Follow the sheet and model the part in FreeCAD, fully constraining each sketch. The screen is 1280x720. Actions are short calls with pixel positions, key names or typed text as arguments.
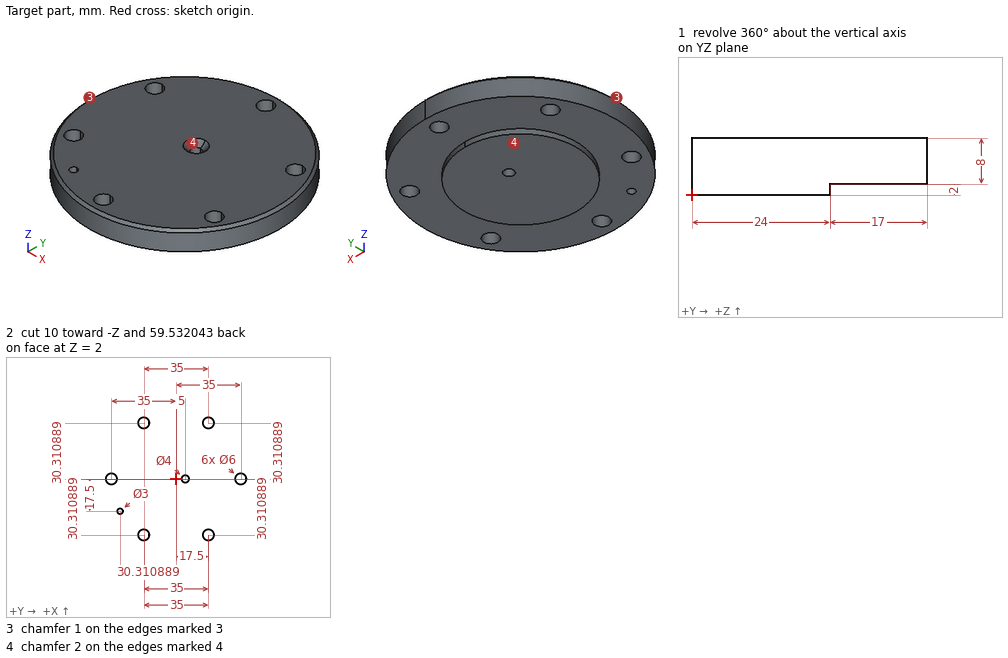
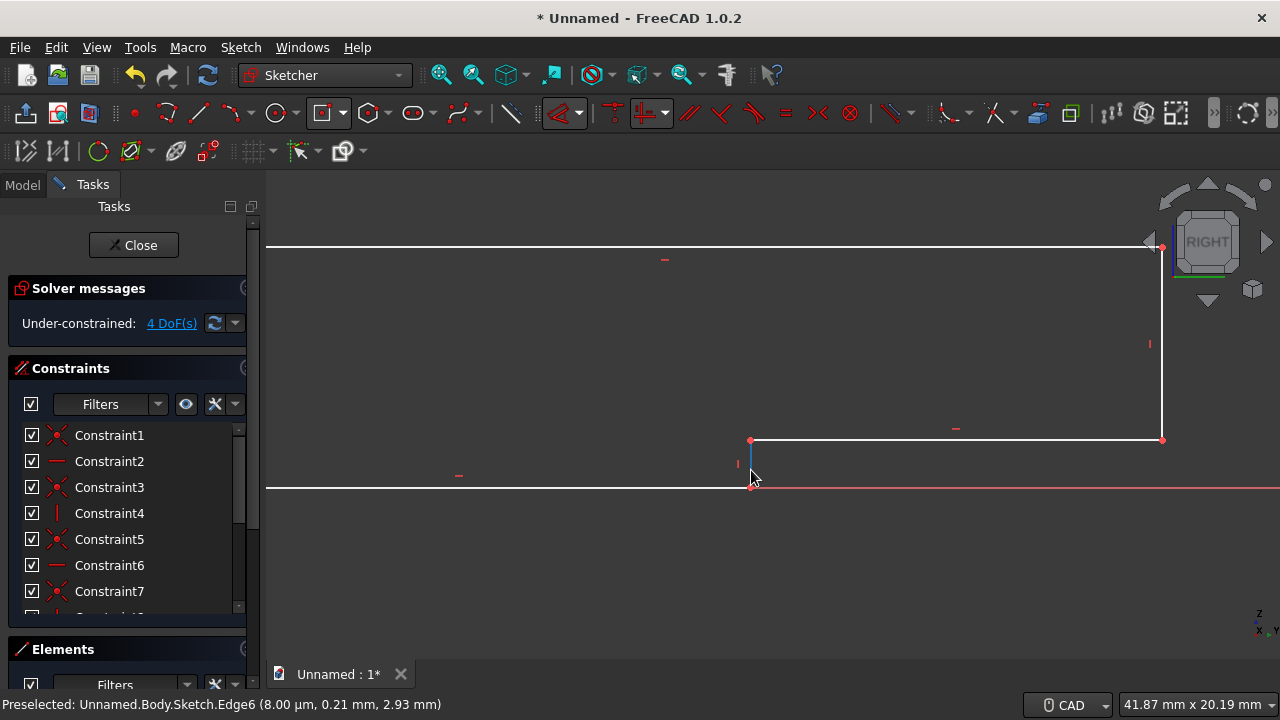
click(751, 469)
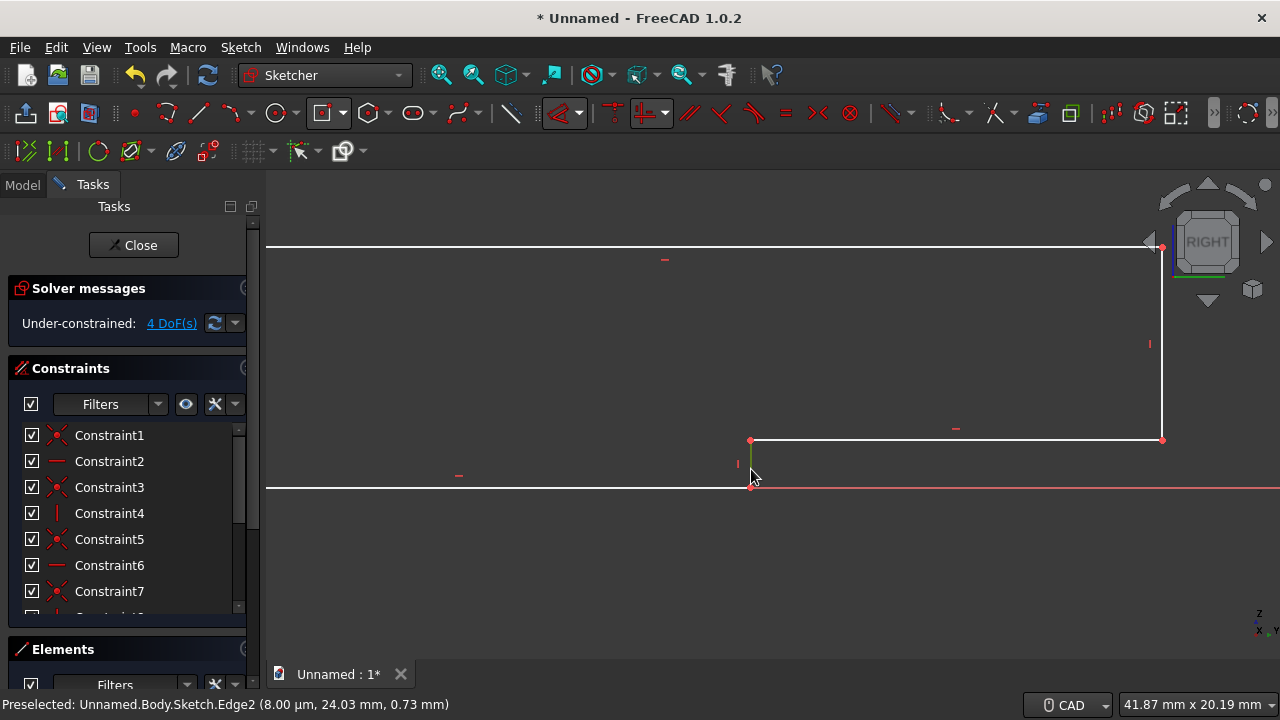
key(i)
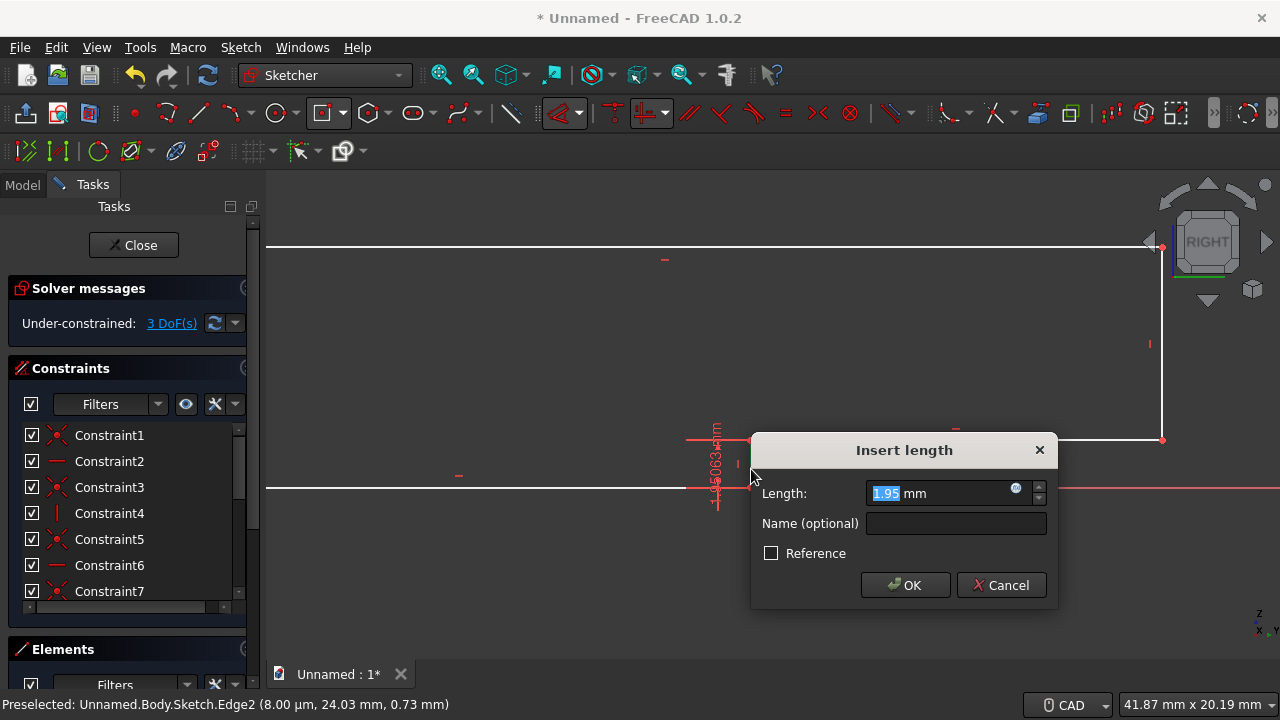
text(2)
key(Return)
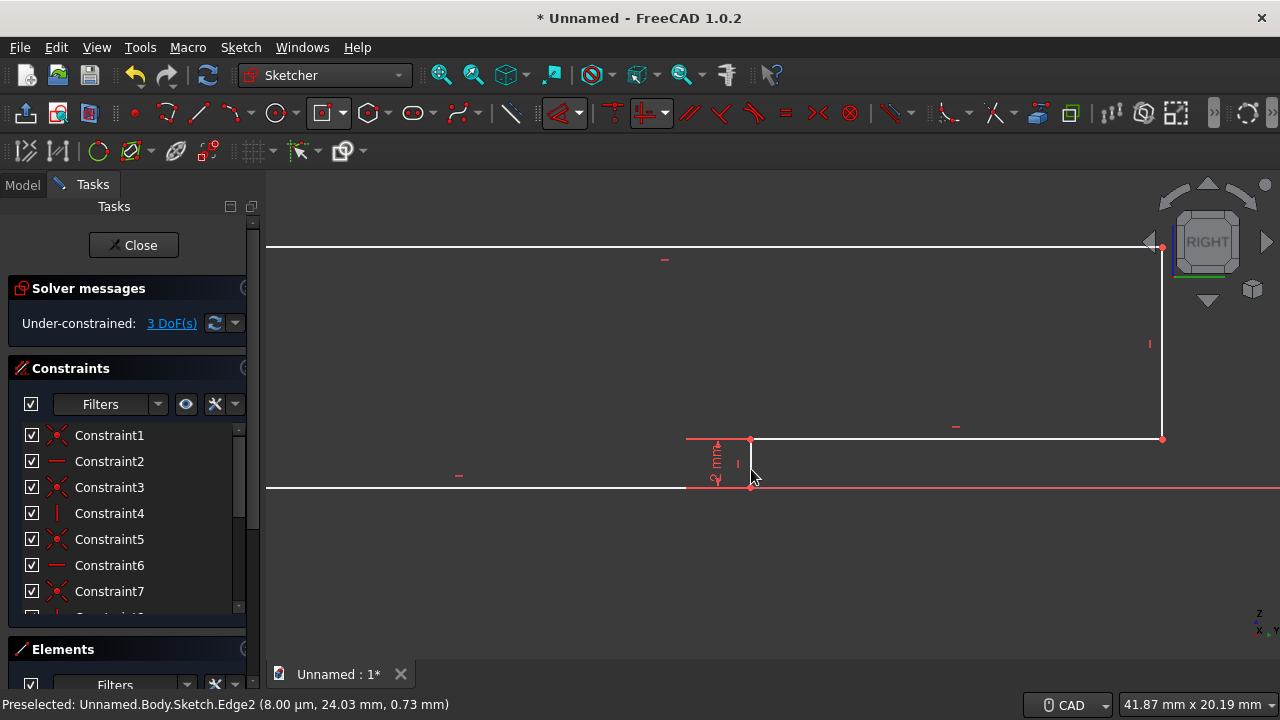
scroll(752, 473, down, 3)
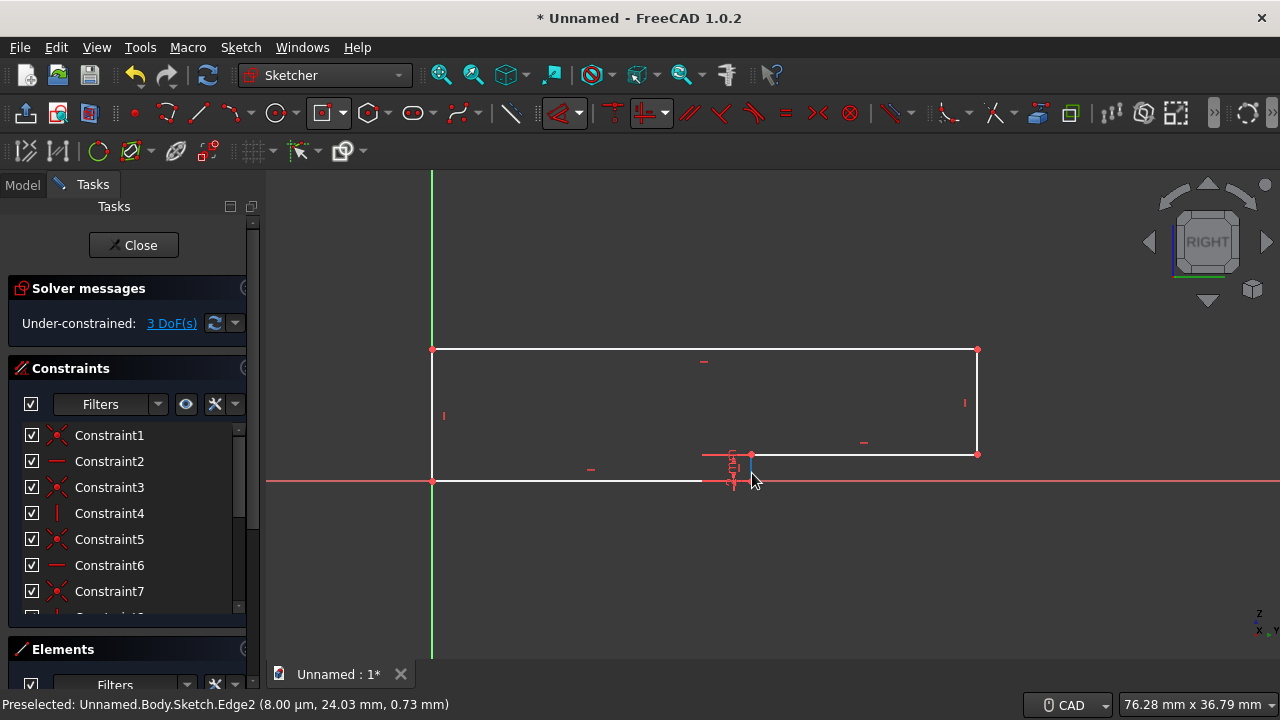
click(977, 423)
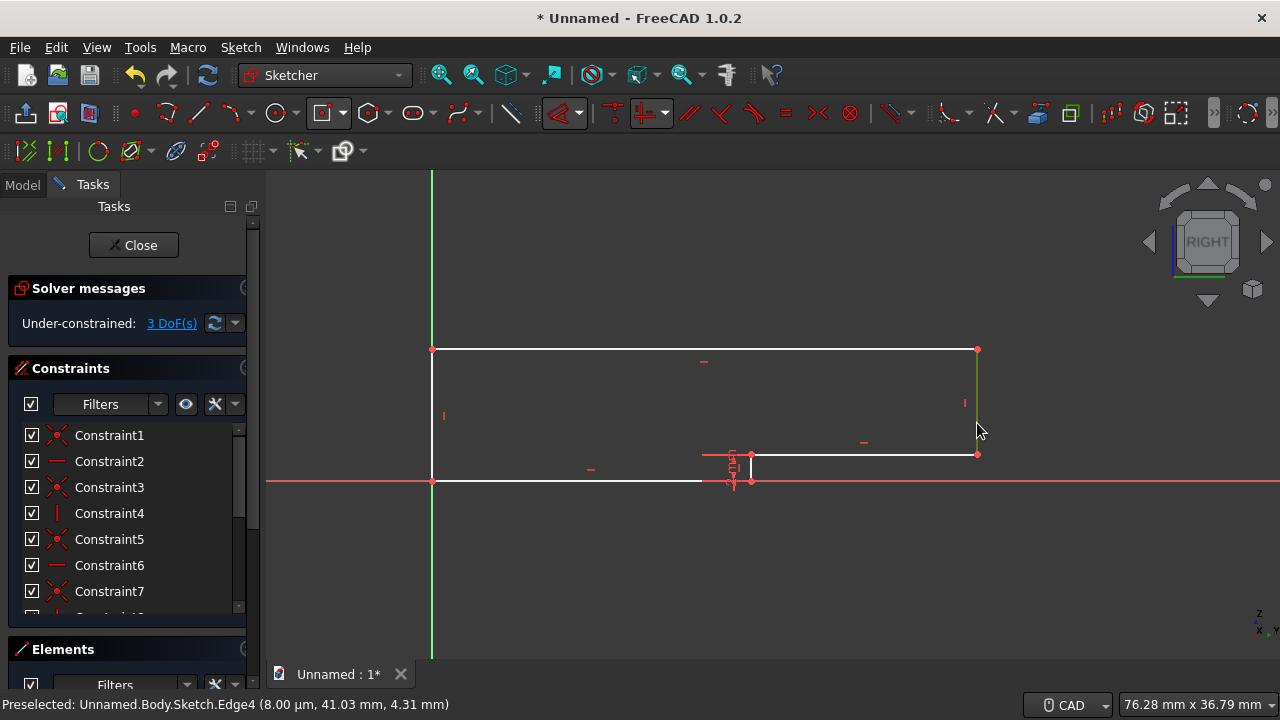
click(582, 114)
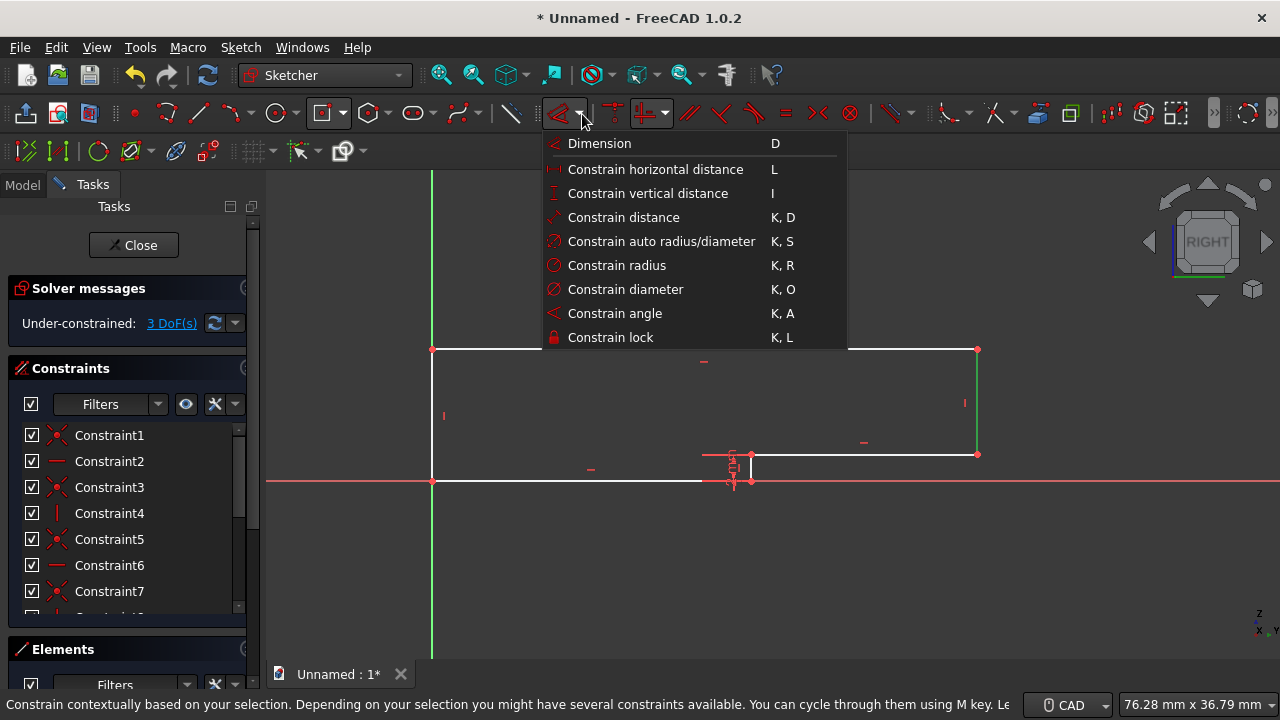
click(695, 193)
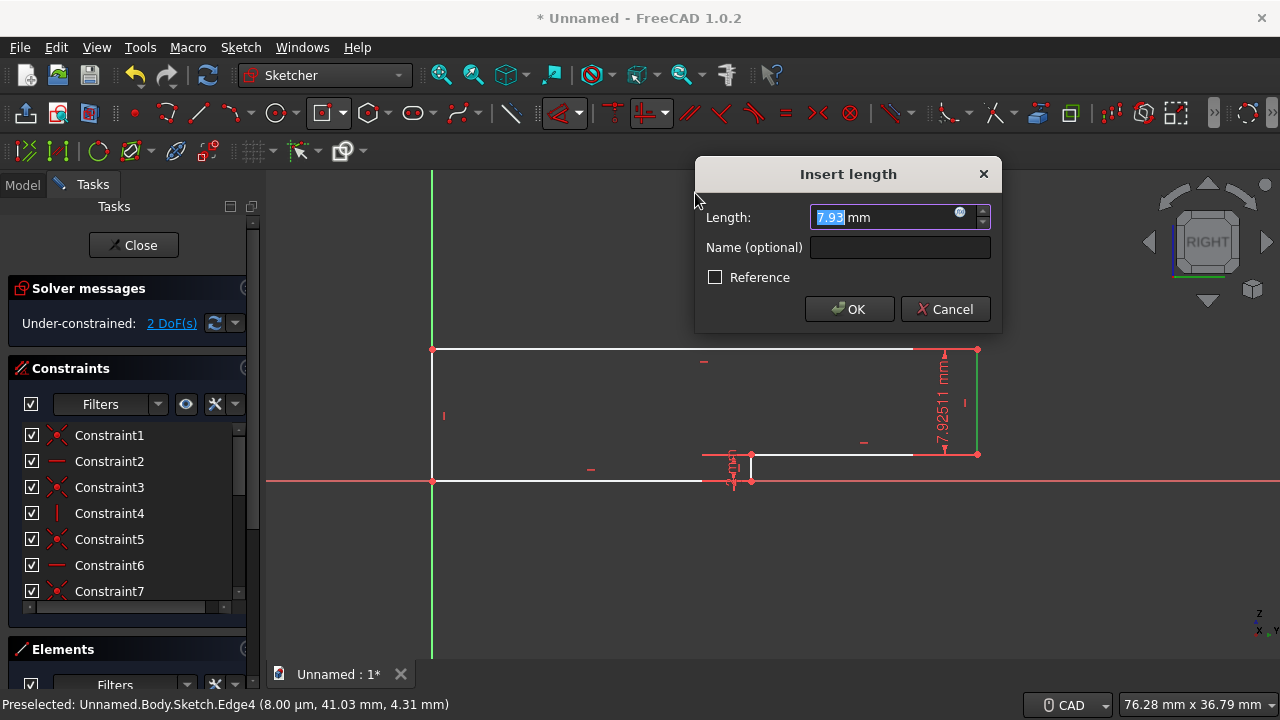
text(8)
key(Return)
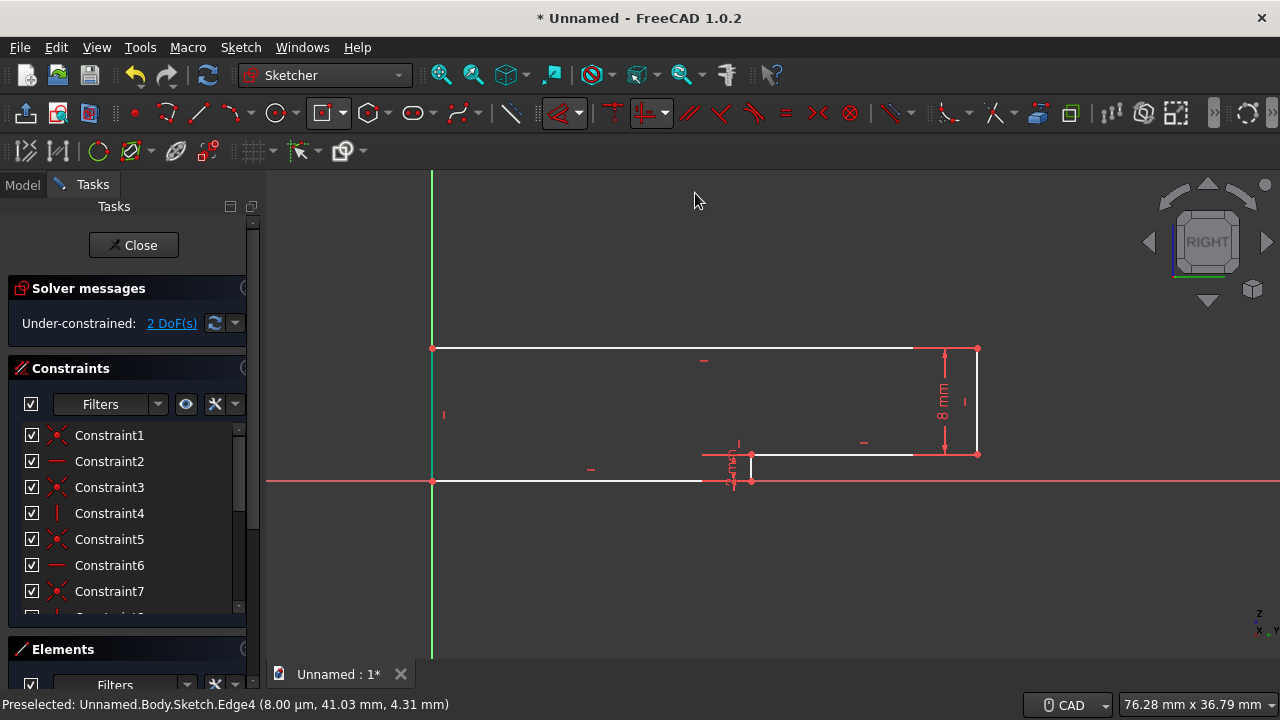
click(528, 481)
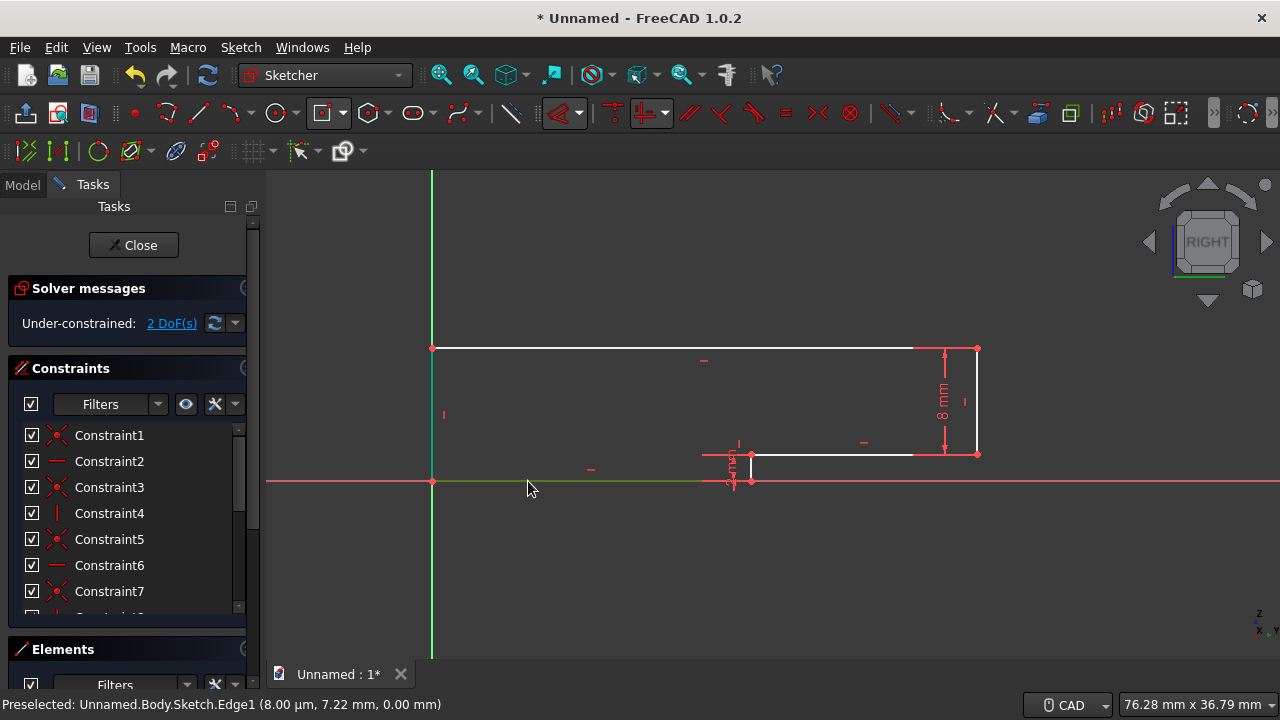
key(l)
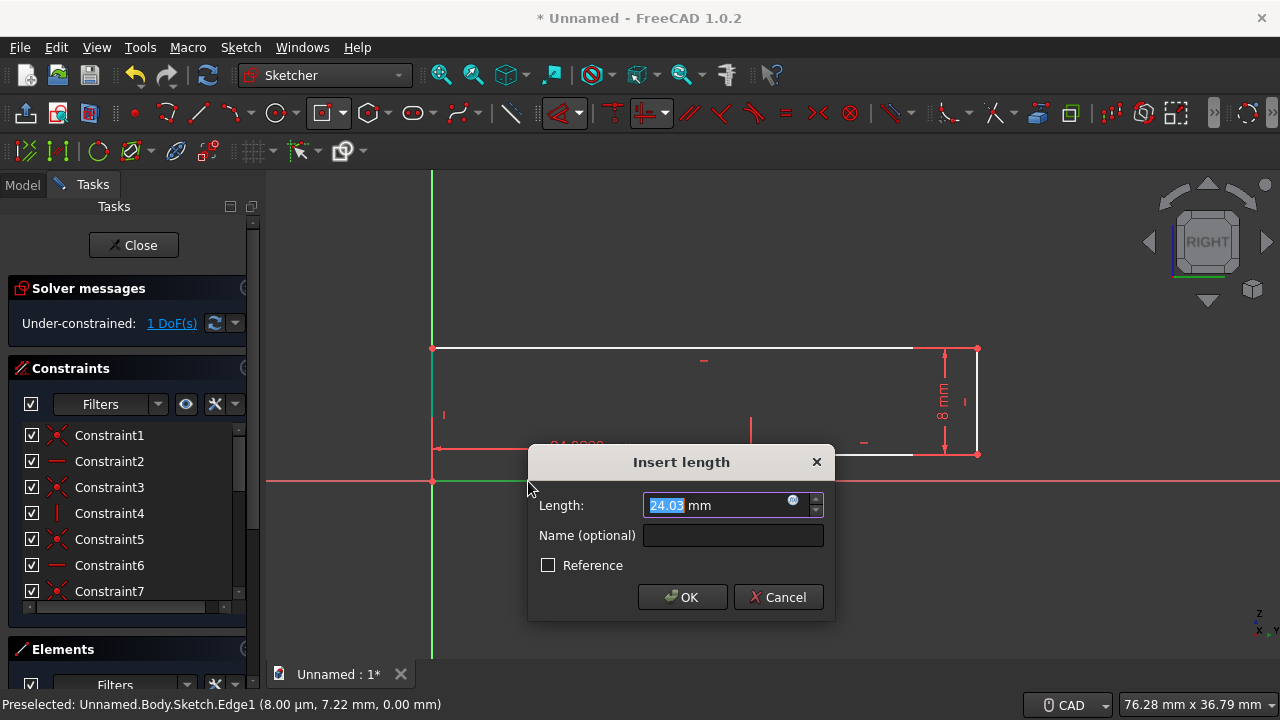
text(24)
key(Return)